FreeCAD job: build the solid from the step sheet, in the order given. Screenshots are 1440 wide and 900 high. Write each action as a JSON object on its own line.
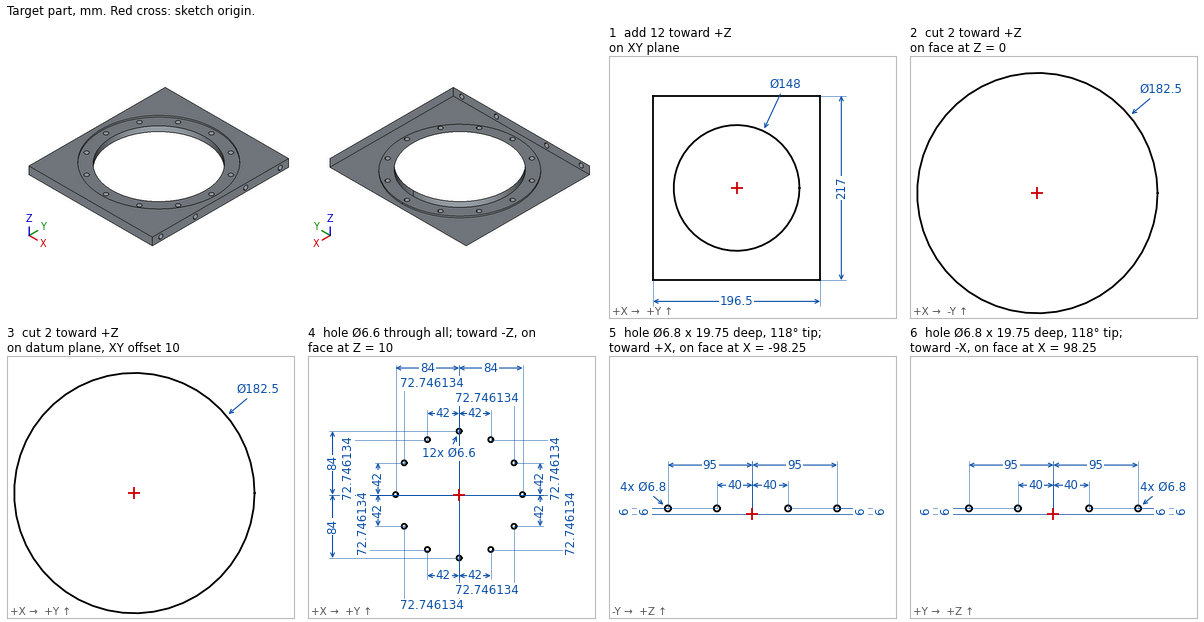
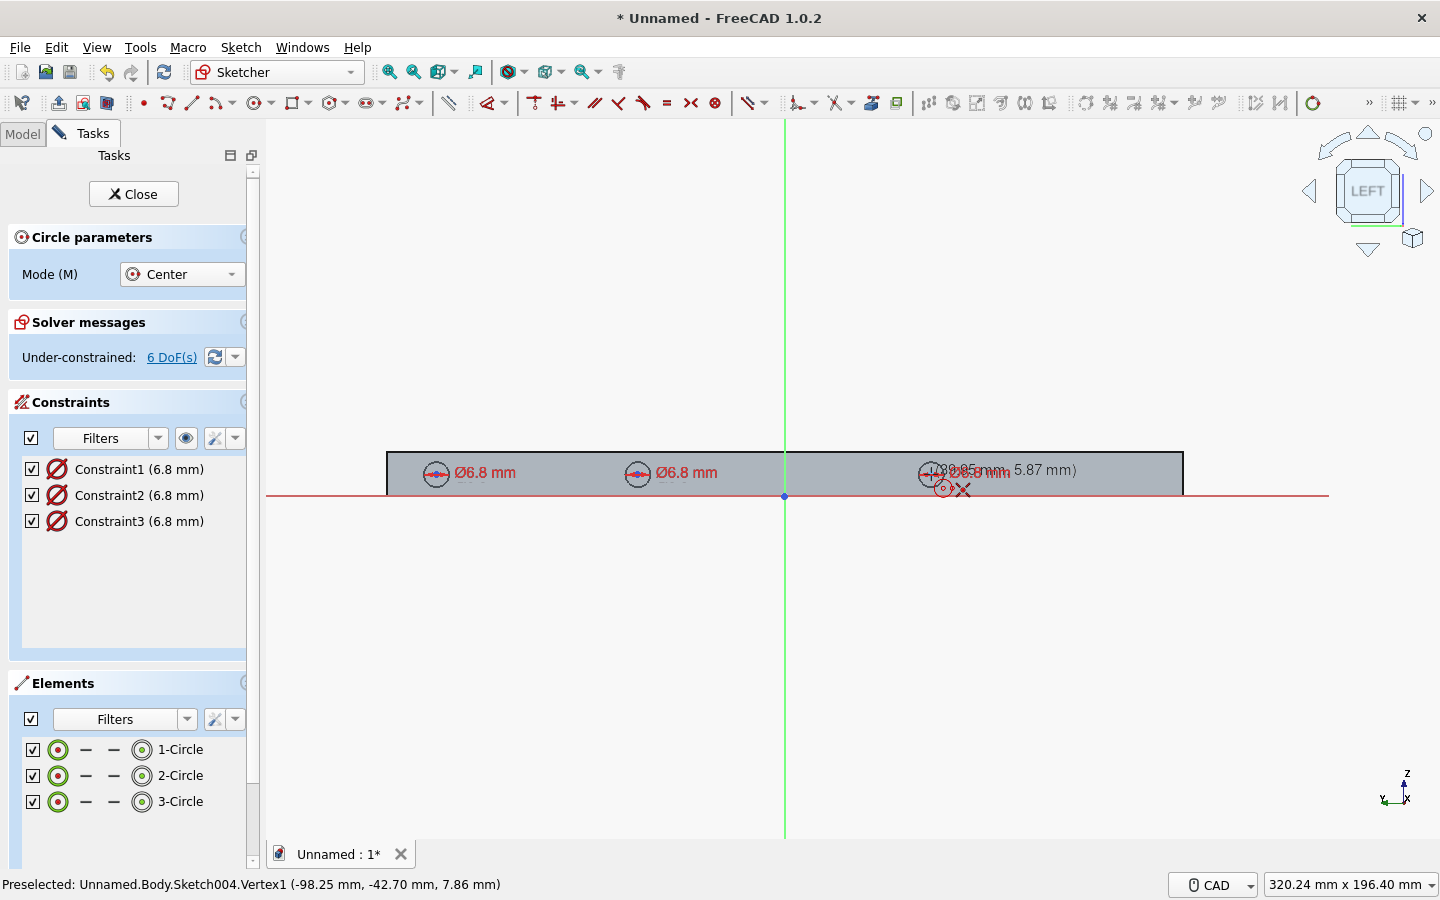
{"action": "scroll", "coordinate": [1133, 474], "scroll_direction": "up", "scroll_amount": 3}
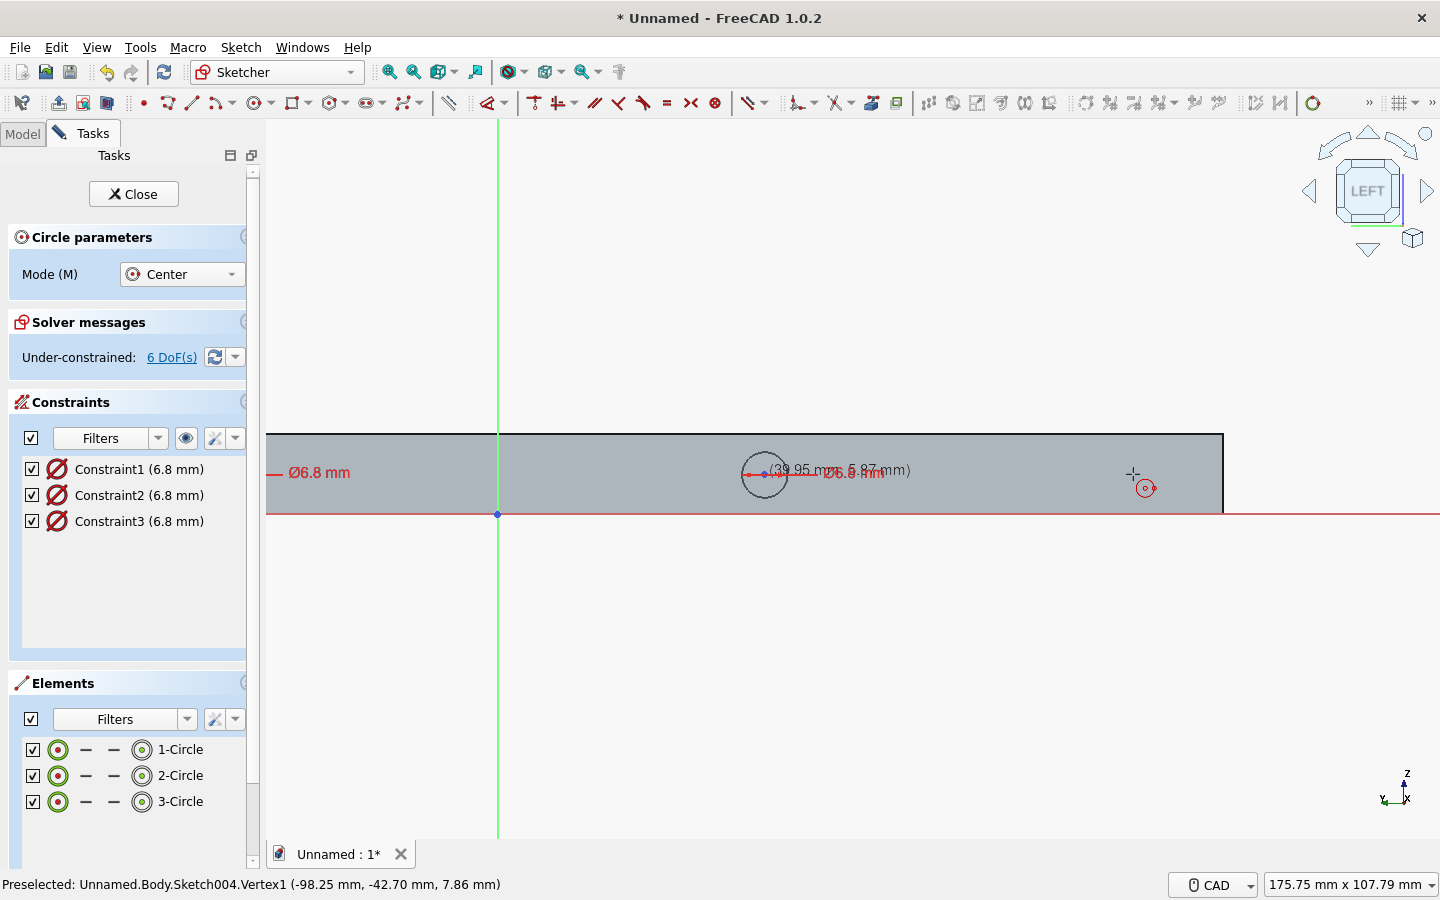
{"action": "left_click", "coordinate": [1132, 474]}
{"action": "mouse_move", "coordinate": [1149, 458]}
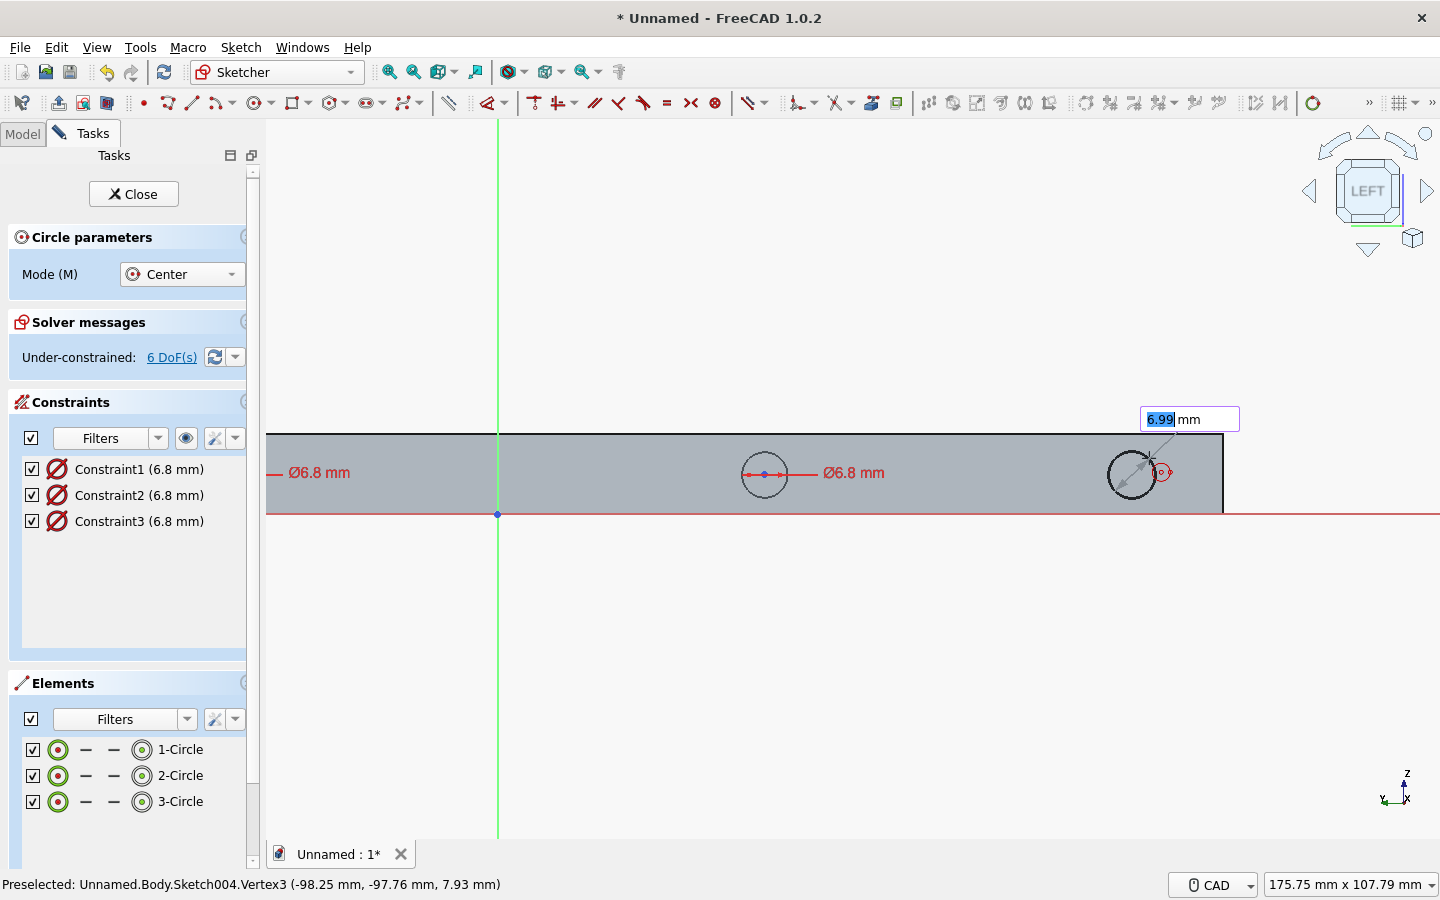
{"action": "type", "text": "6.8"}
{"action": "key", "text": "Return"}
{"action": "key", "text": "Escape"}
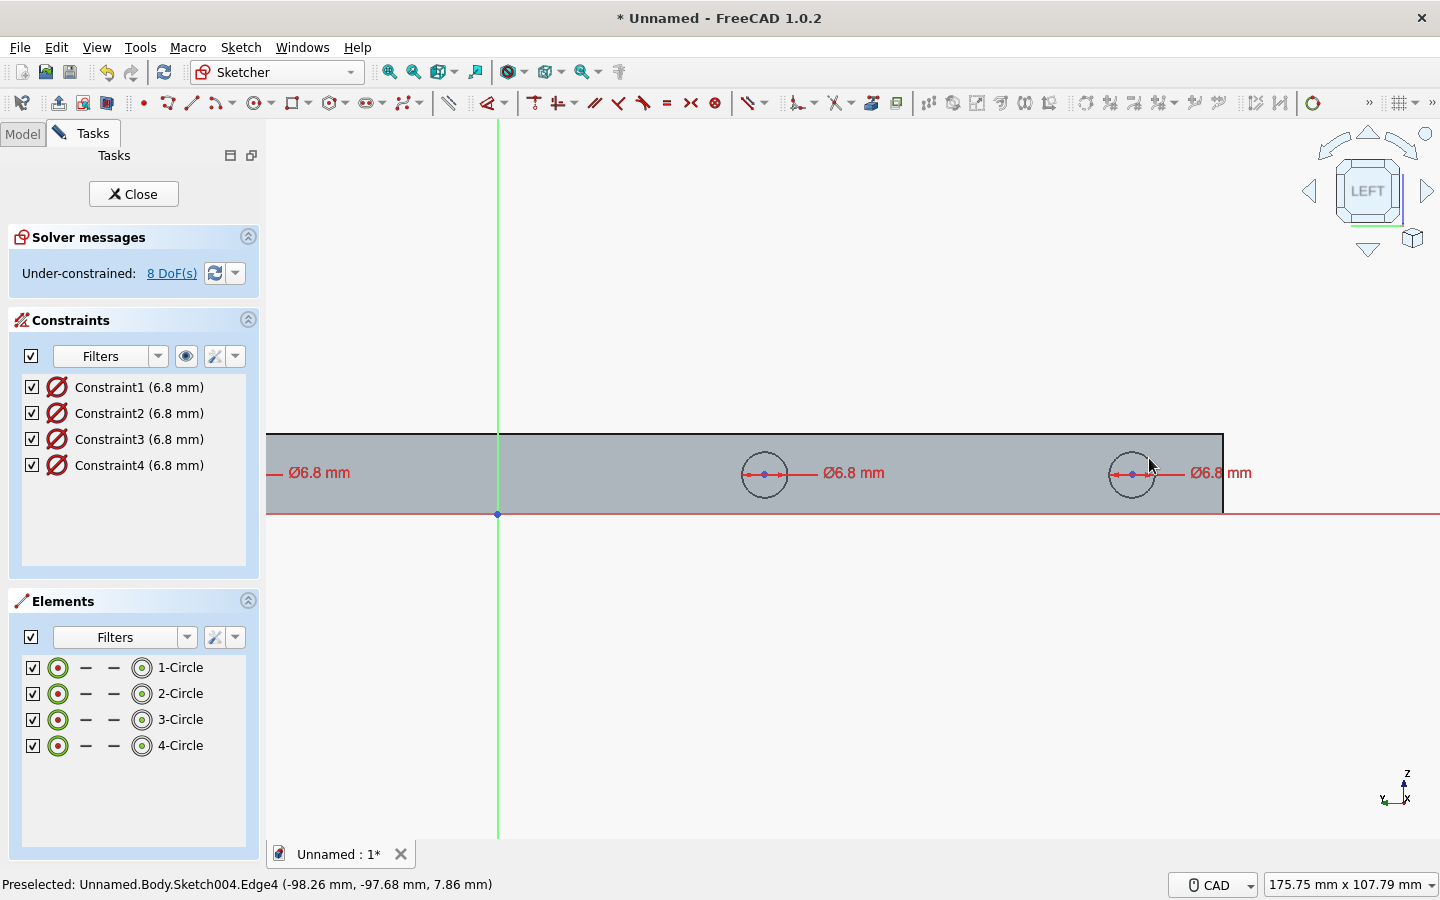
{"action": "left_click", "coordinate": [488, 104]}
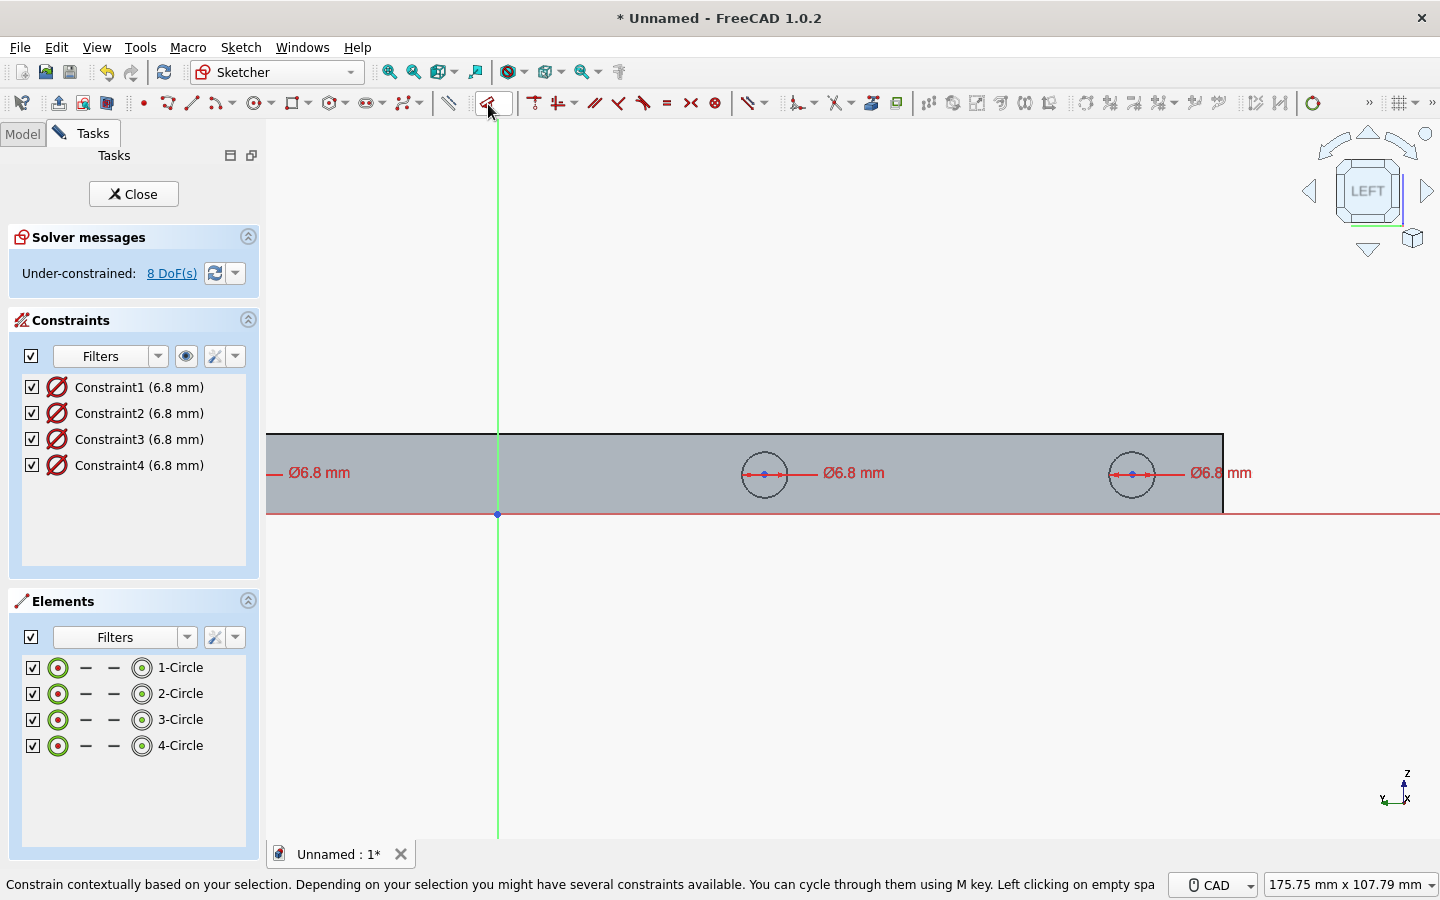
{"action": "scroll", "coordinate": [1133, 474], "scroll_direction": "down", "scroll_amount": 3}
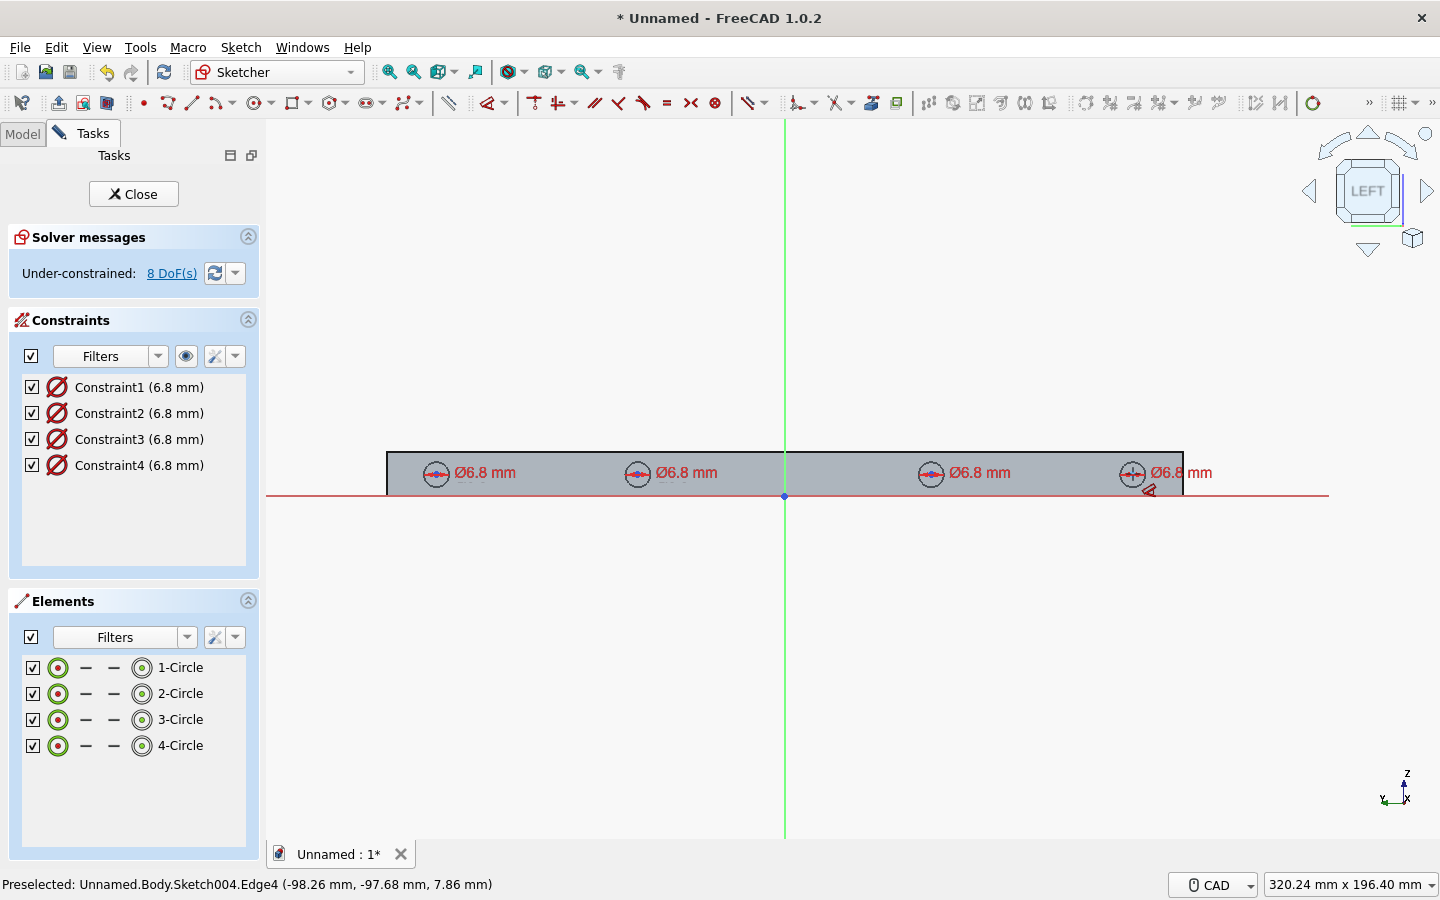
{"action": "scroll", "coordinate": [437, 475], "scroll_direction": "up", "scroll_amount": 3}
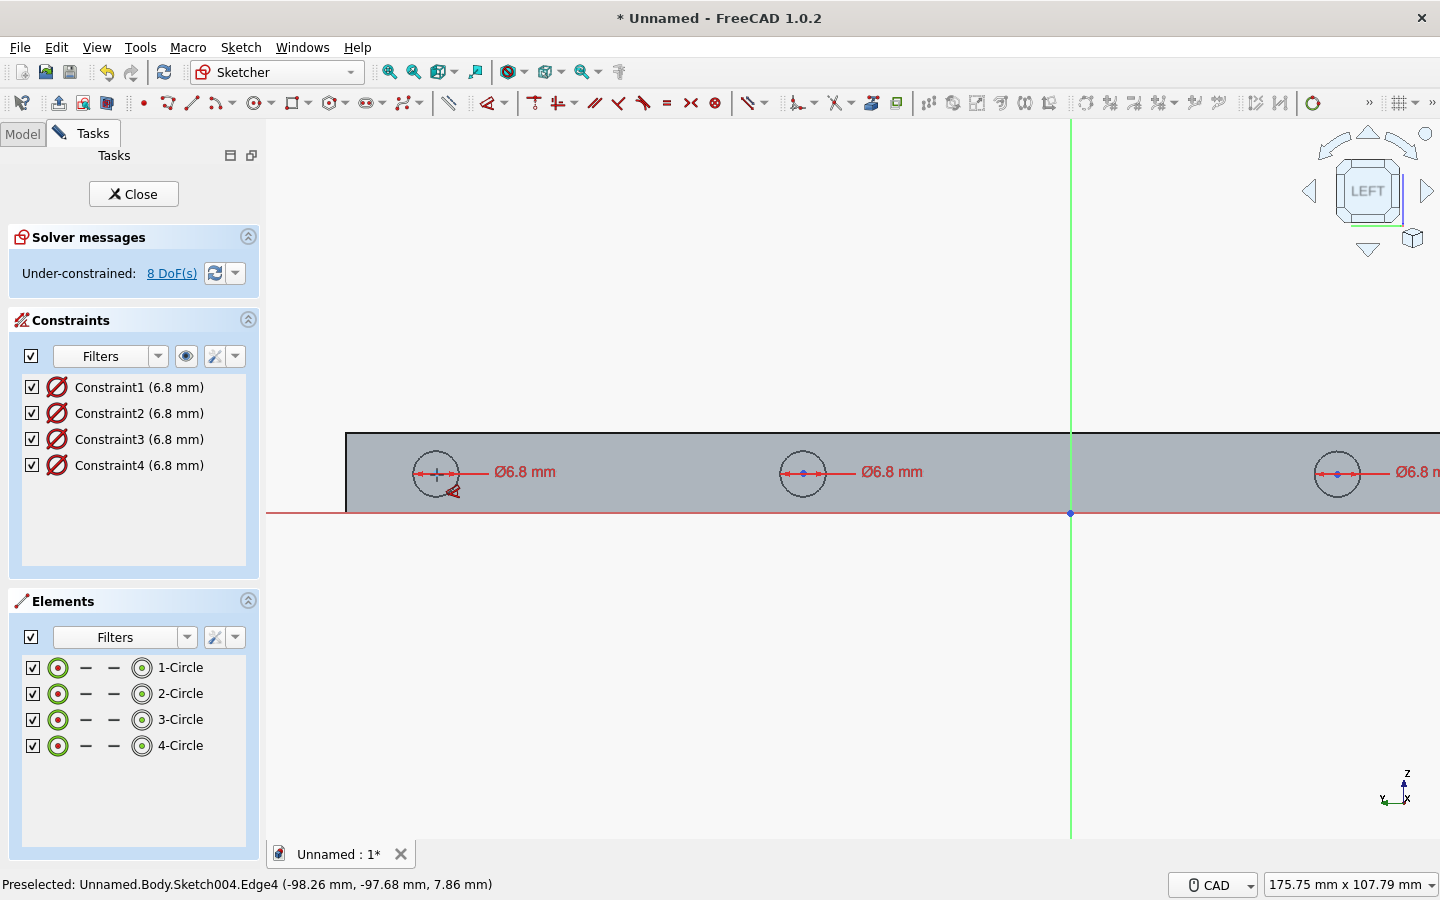
{"action": "left_click", "coordinate": [436, 474]}
{"action": "left_click", "coordinate": [402, 494]}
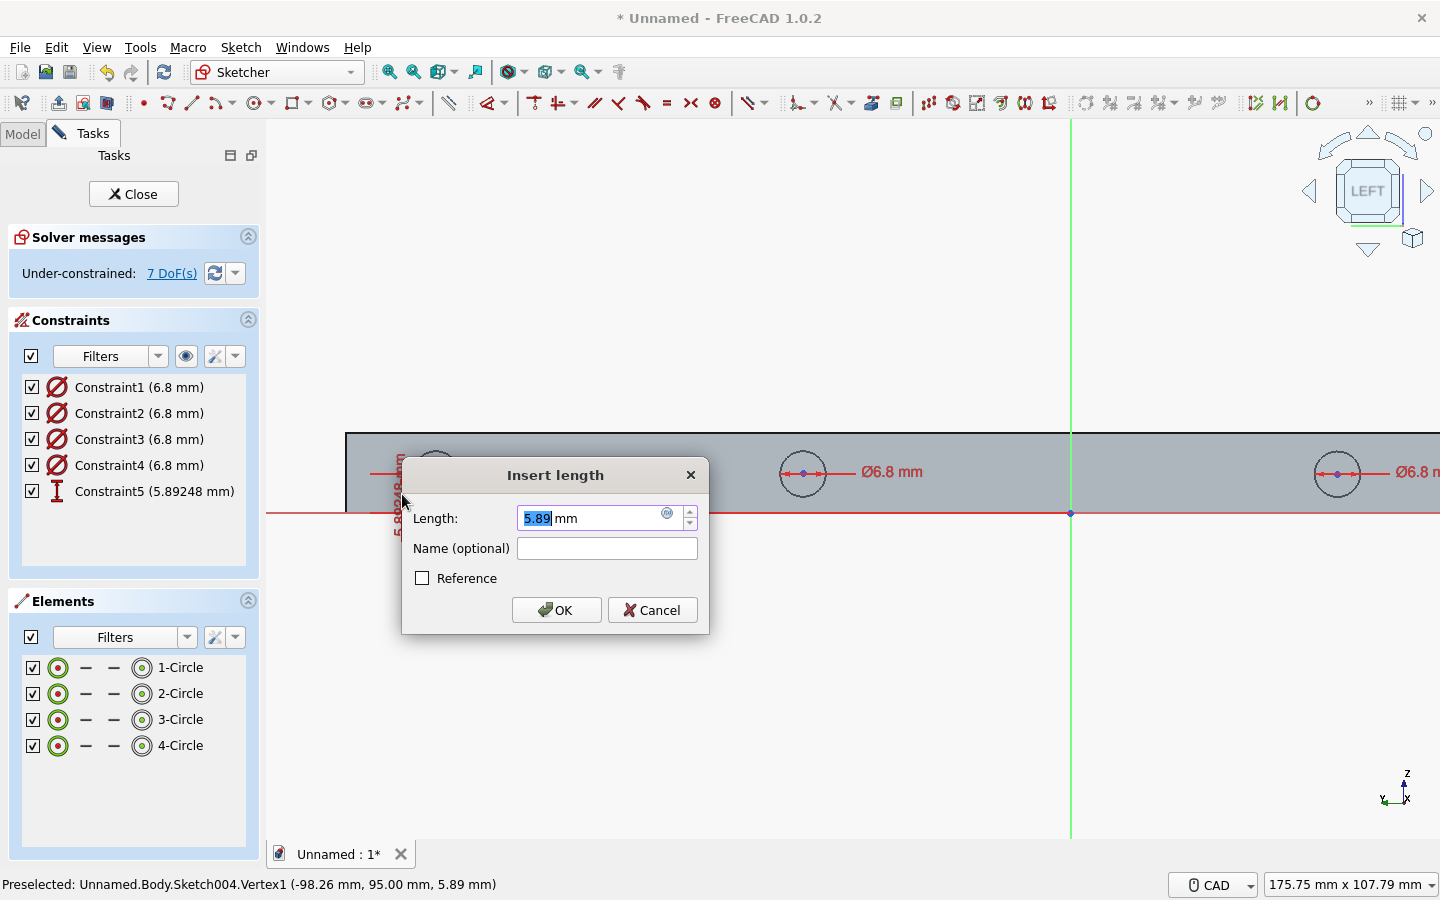
{"action": "type", "text": "6"}
{"action": "key", "text": "Return"}